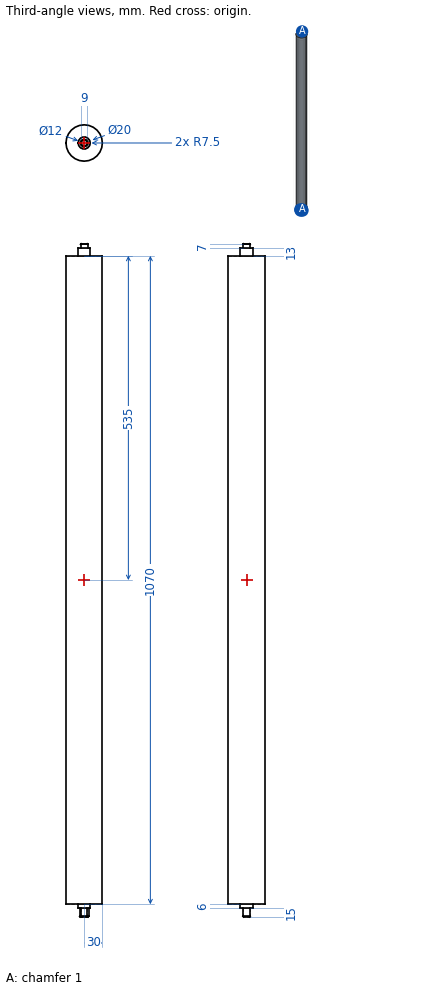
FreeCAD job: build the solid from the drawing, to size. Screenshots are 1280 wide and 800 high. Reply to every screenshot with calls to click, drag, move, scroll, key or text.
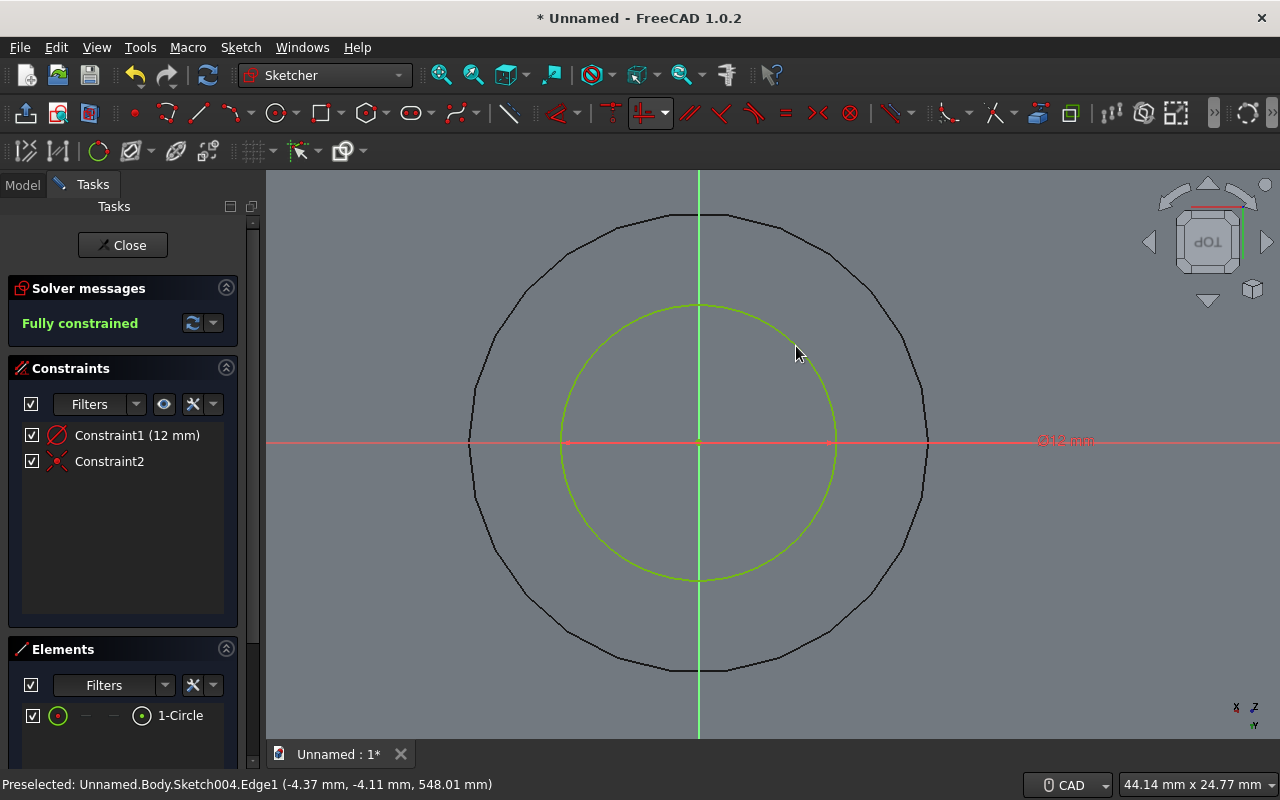
click(123, 245)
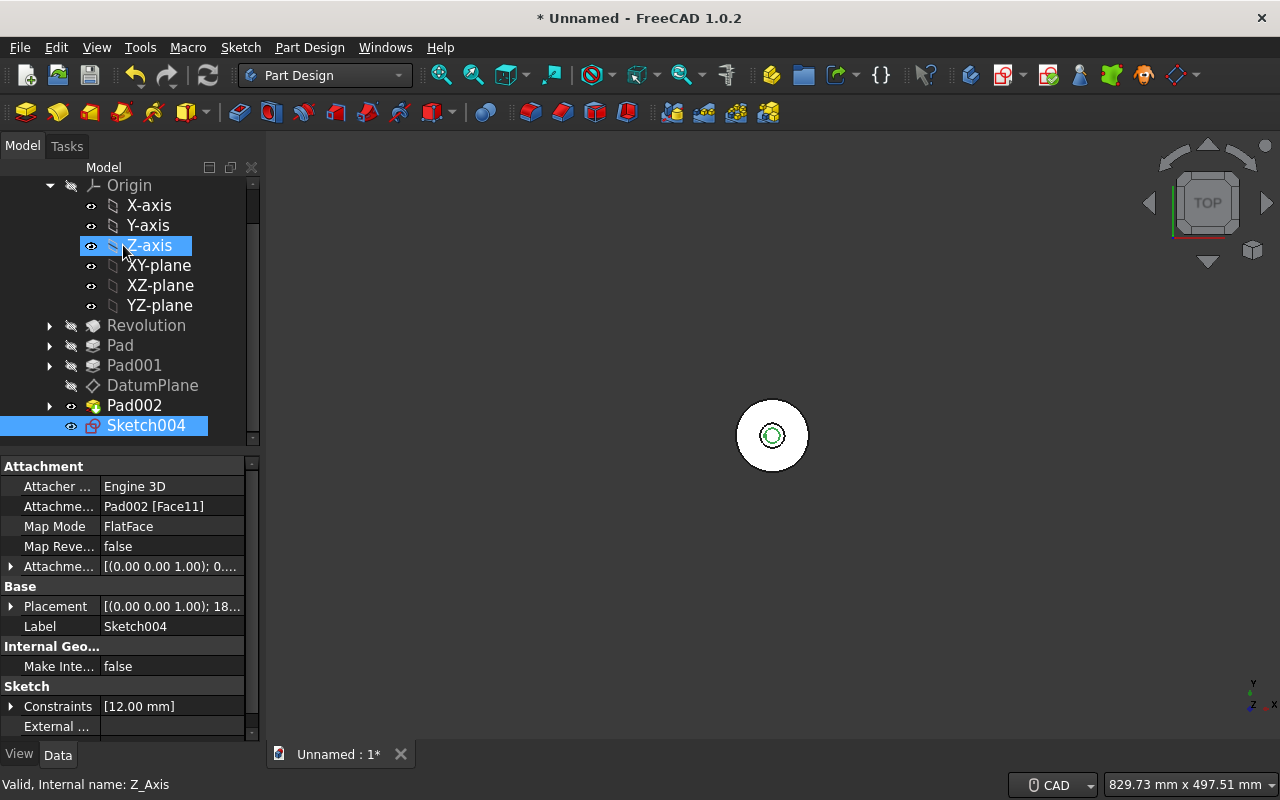
click(26, 112)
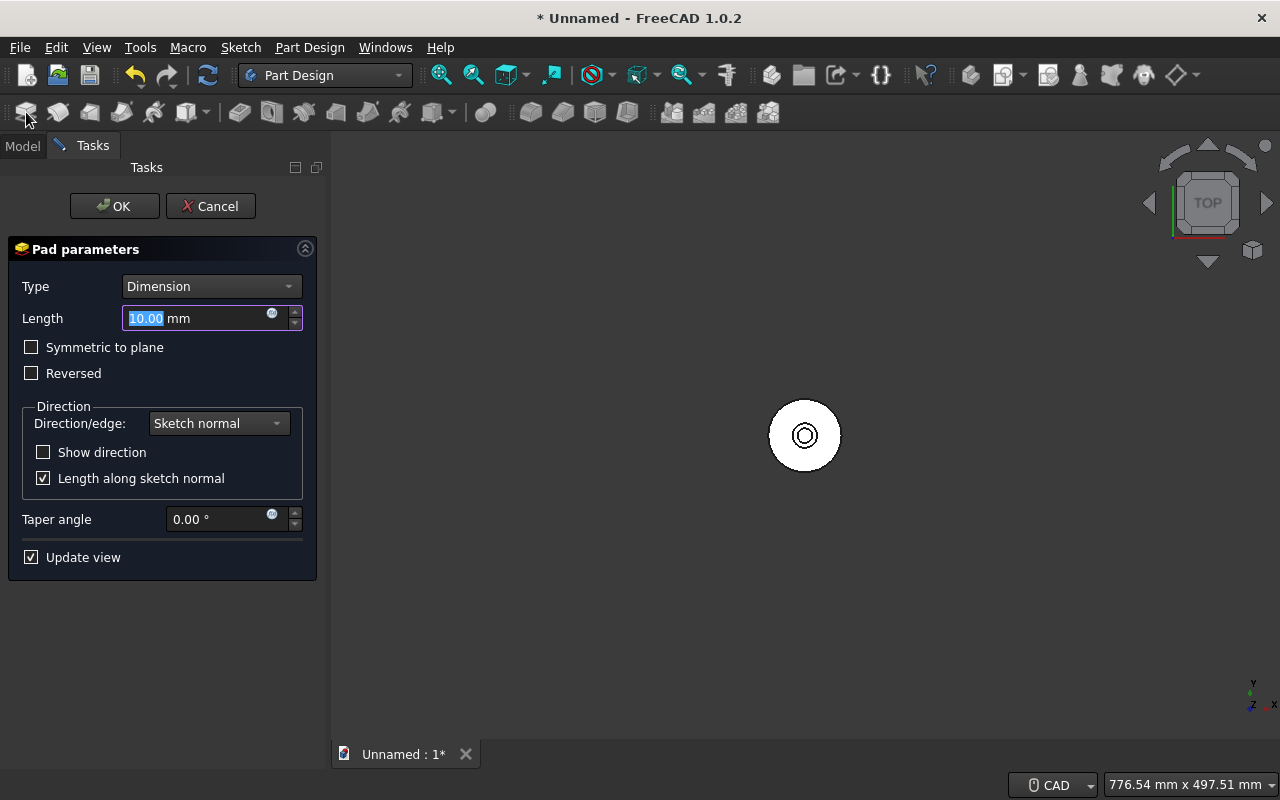
text(7)
key(Tab)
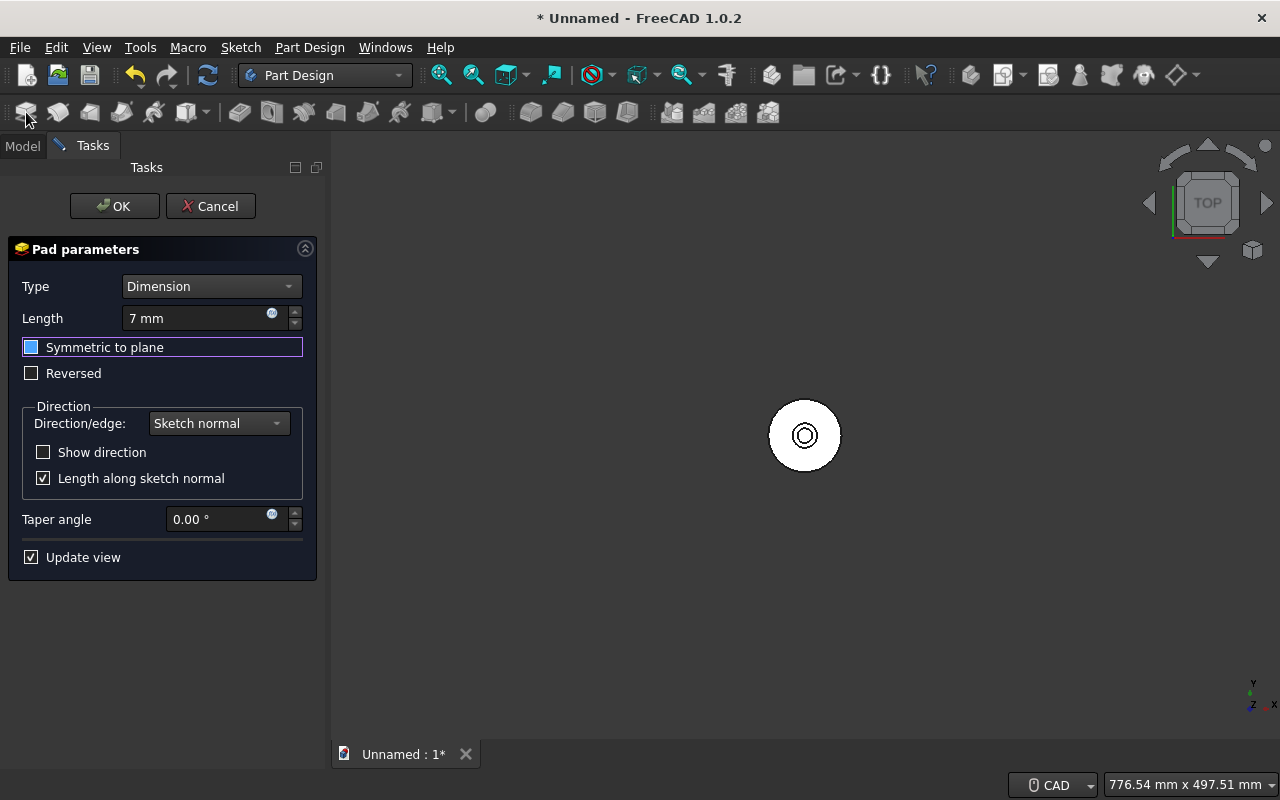
click(115, 206)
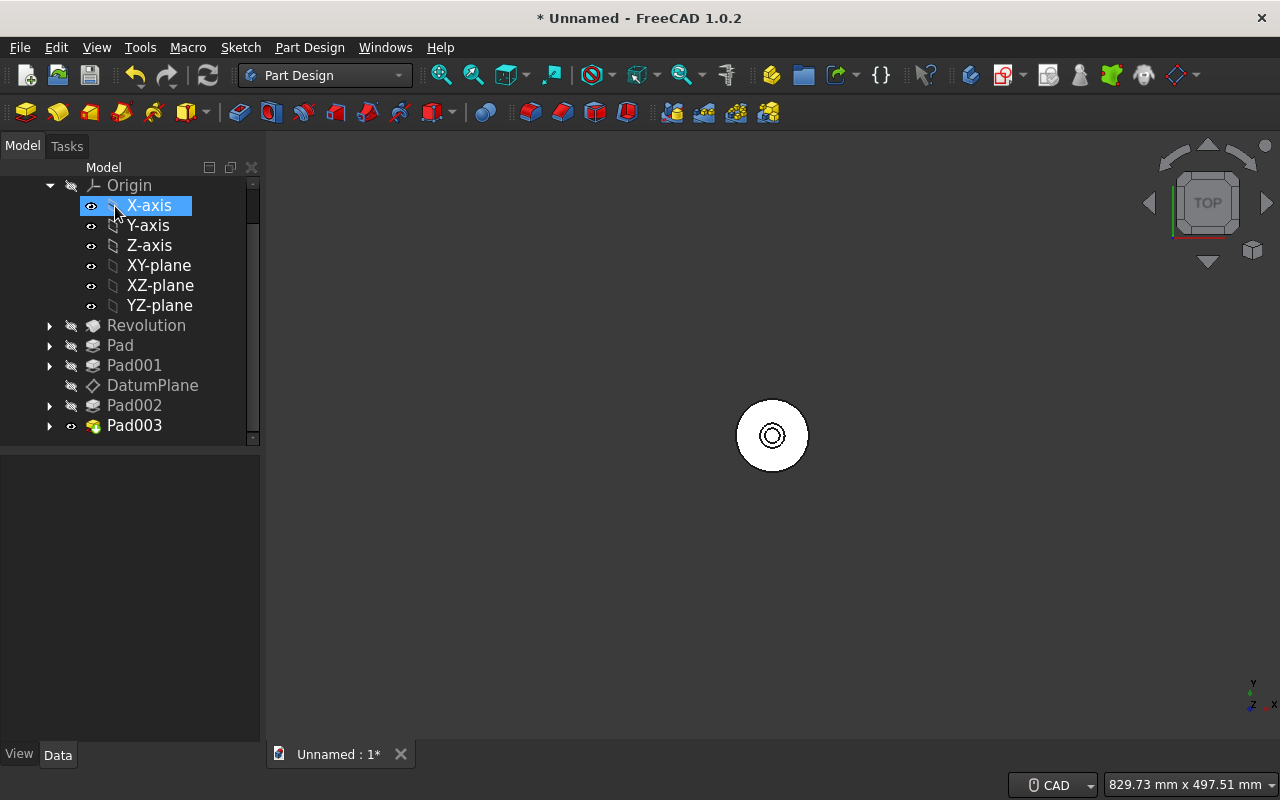
click(442, 76)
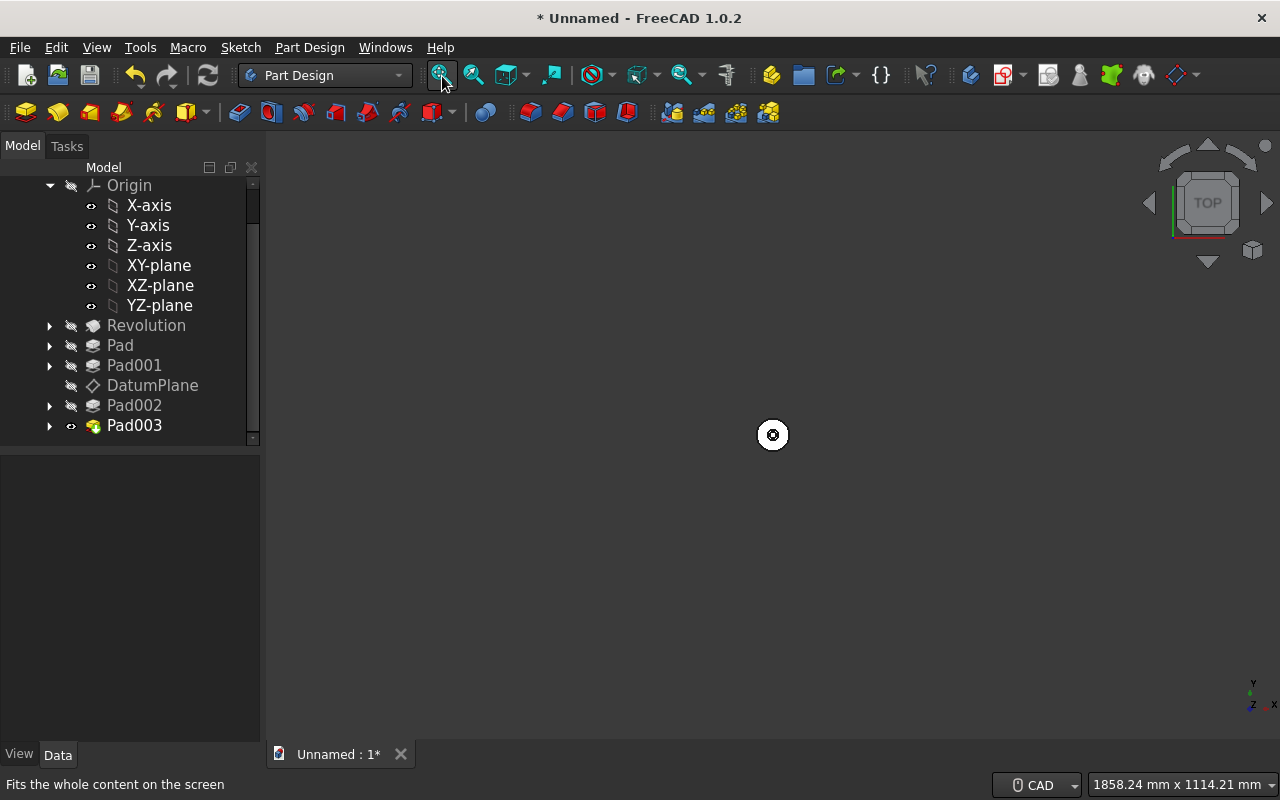
click(776, 434)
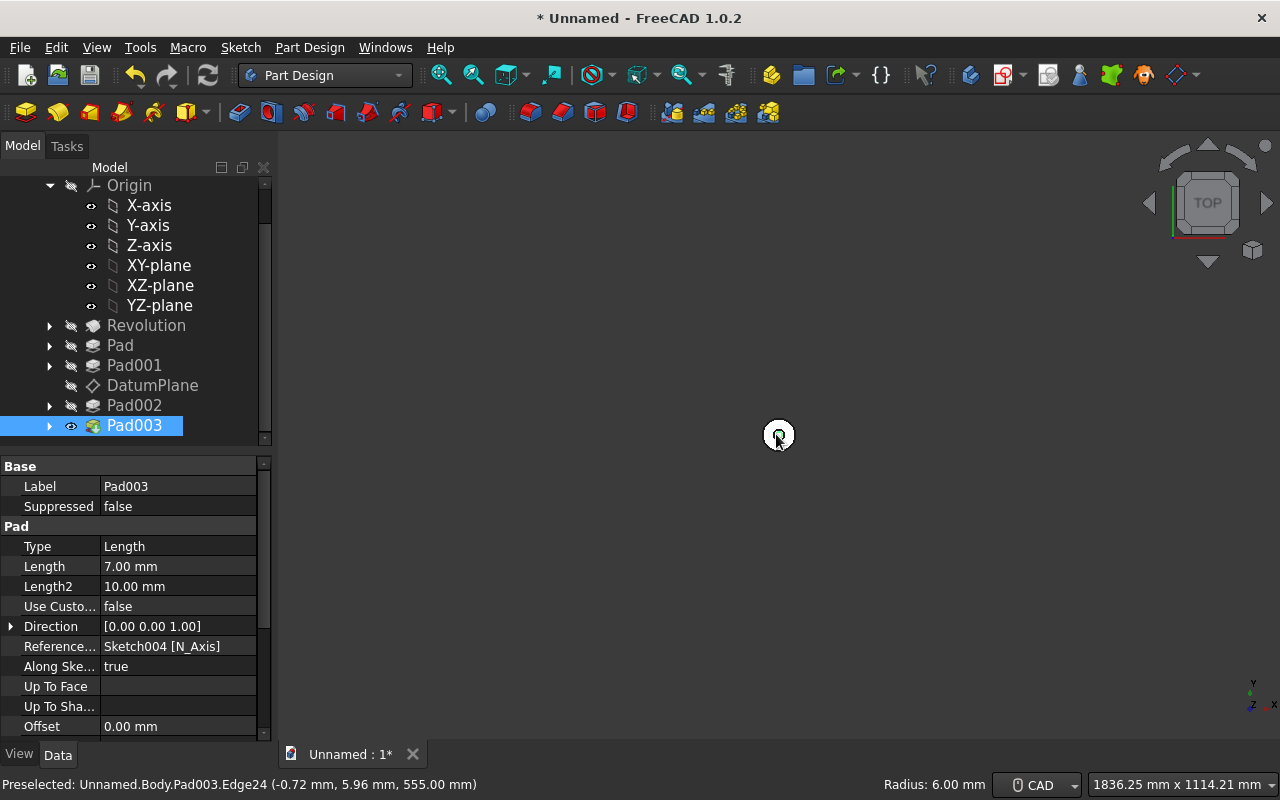
scroll(779, 434, up, 7)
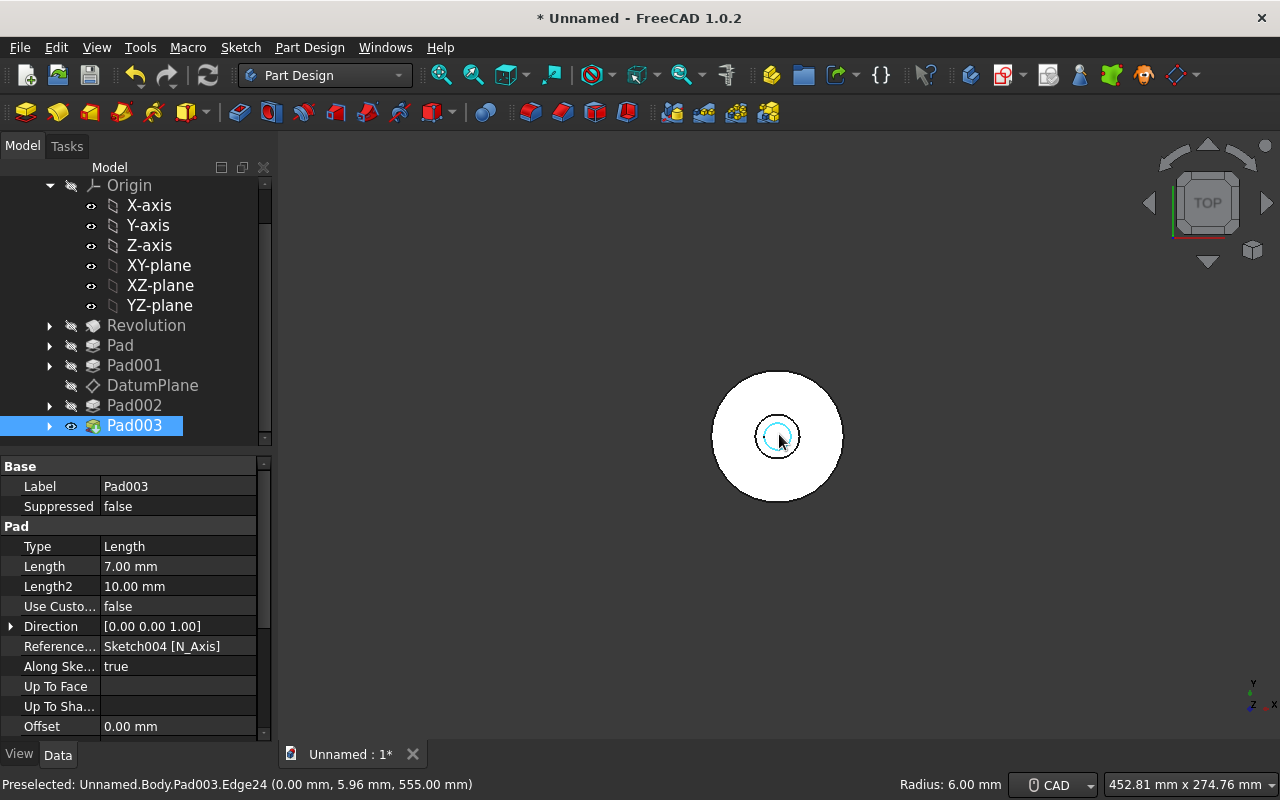
key(v)
key(f)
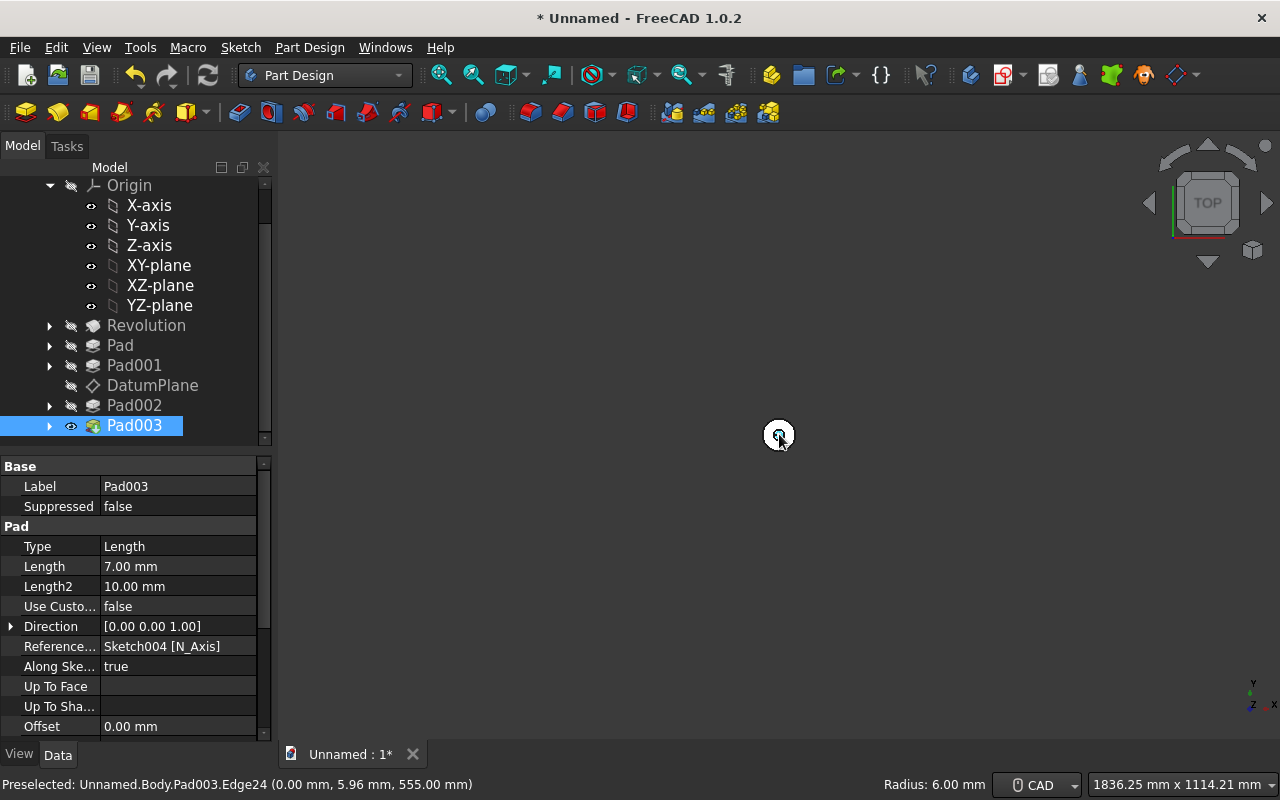
key(0)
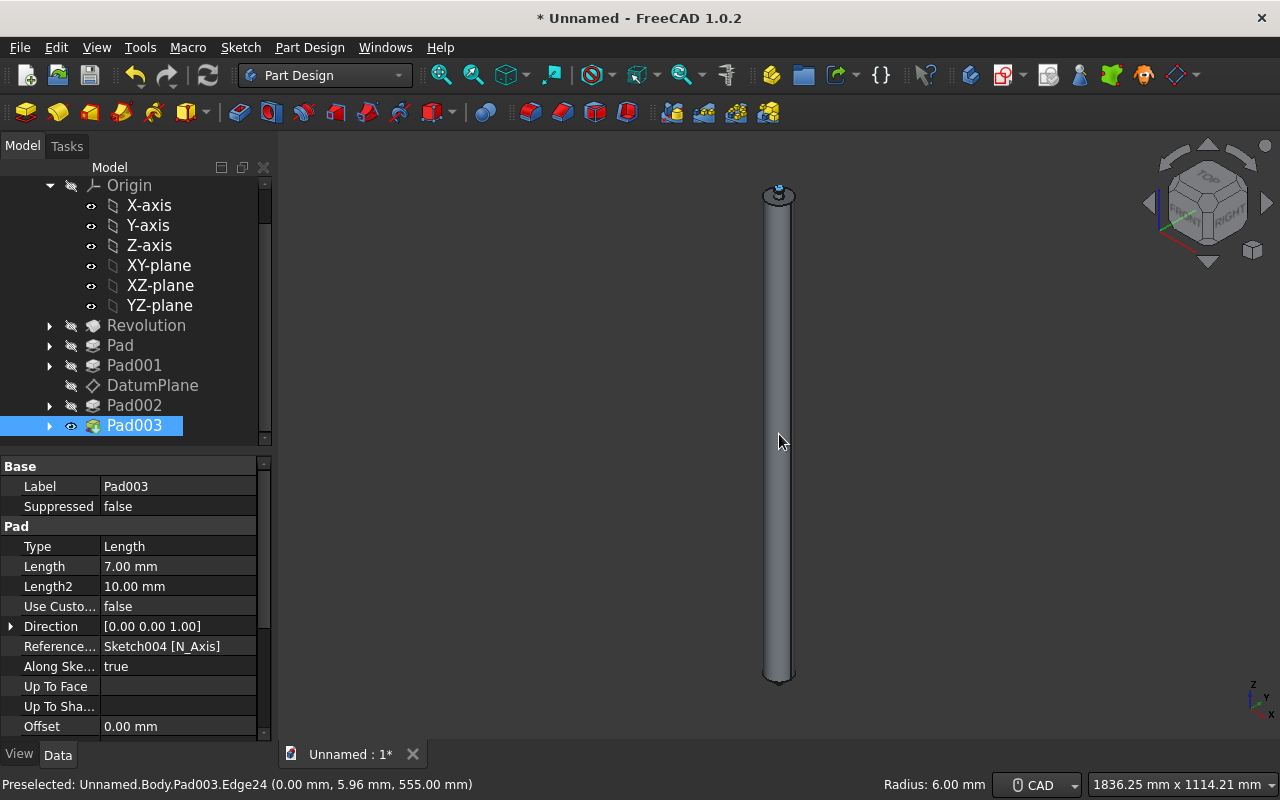
scroll(779, 681, up, 7)